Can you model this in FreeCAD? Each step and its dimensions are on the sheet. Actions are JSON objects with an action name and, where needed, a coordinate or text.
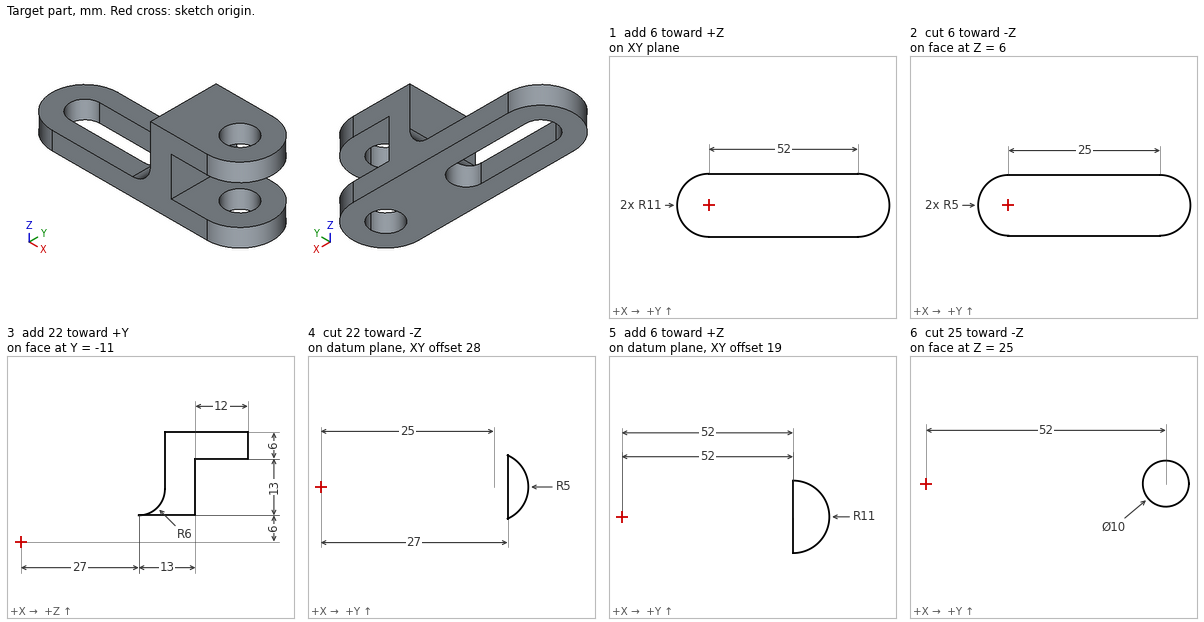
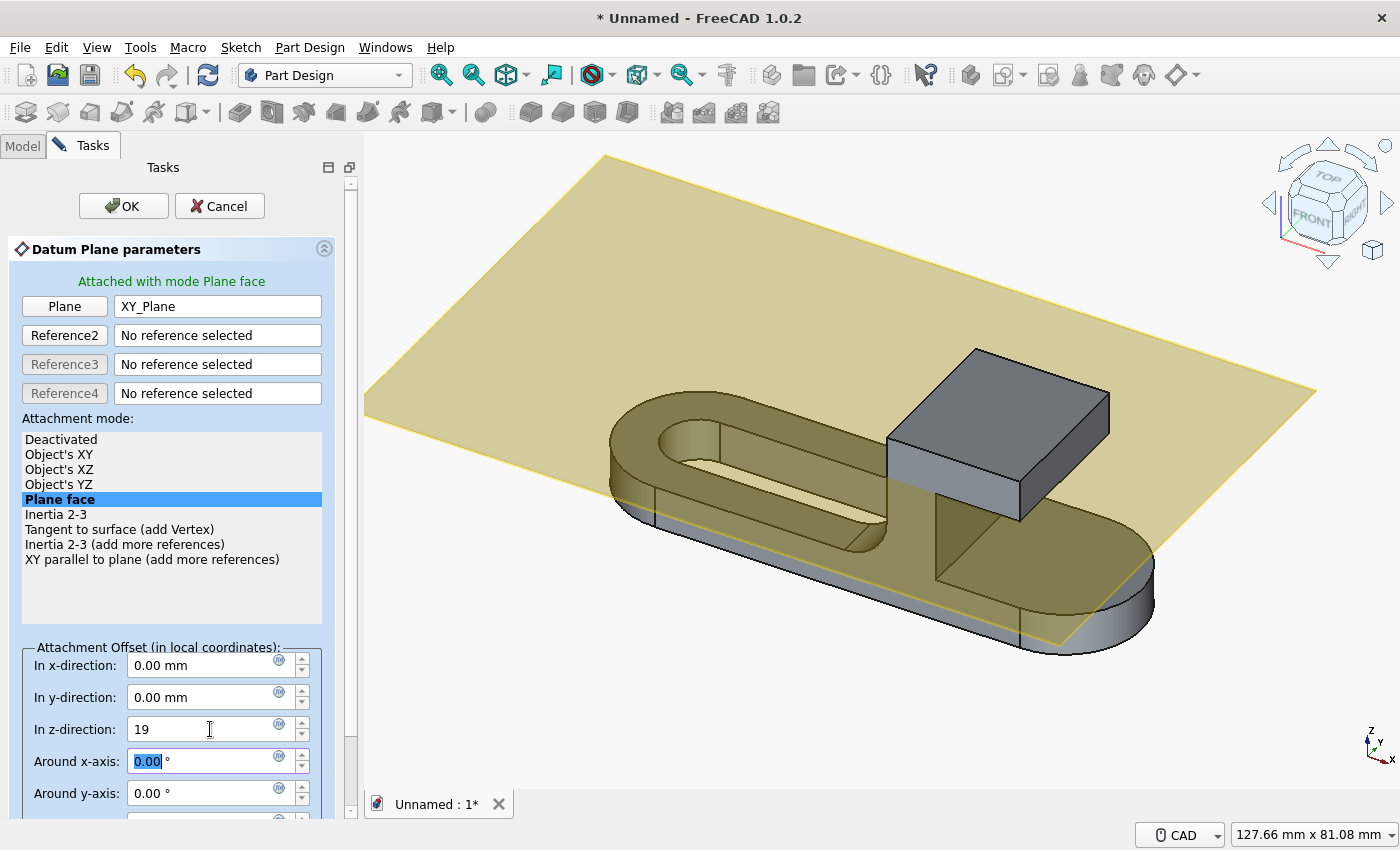
{"action": "left_click", "coordinate": [124, 206]}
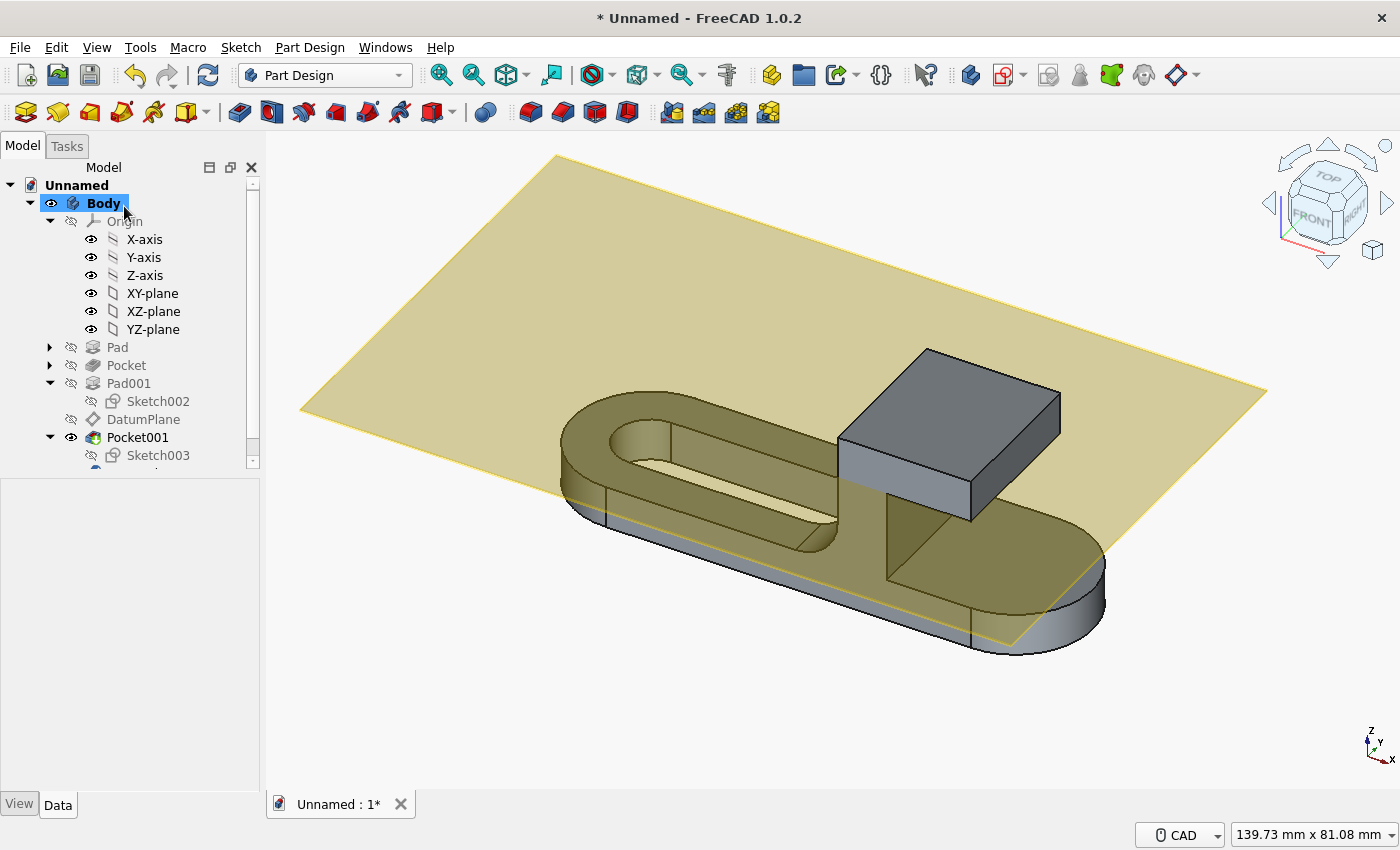
{"action": "scroll", "coordinate": [100, 325], "scroll_direction": "down", "scroll_amount": 3}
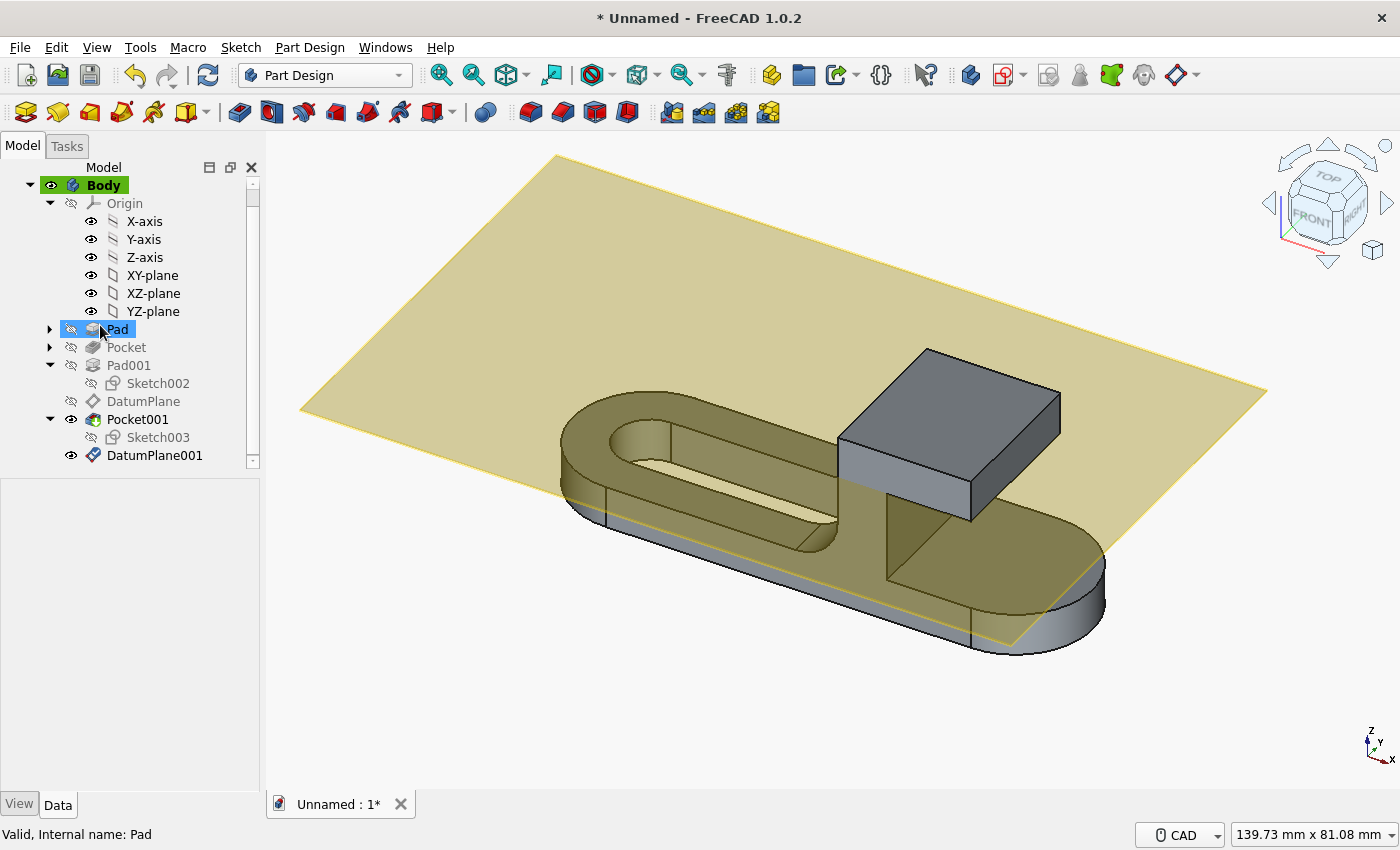
{"action": "left_click", "coordinate": [116, 455]}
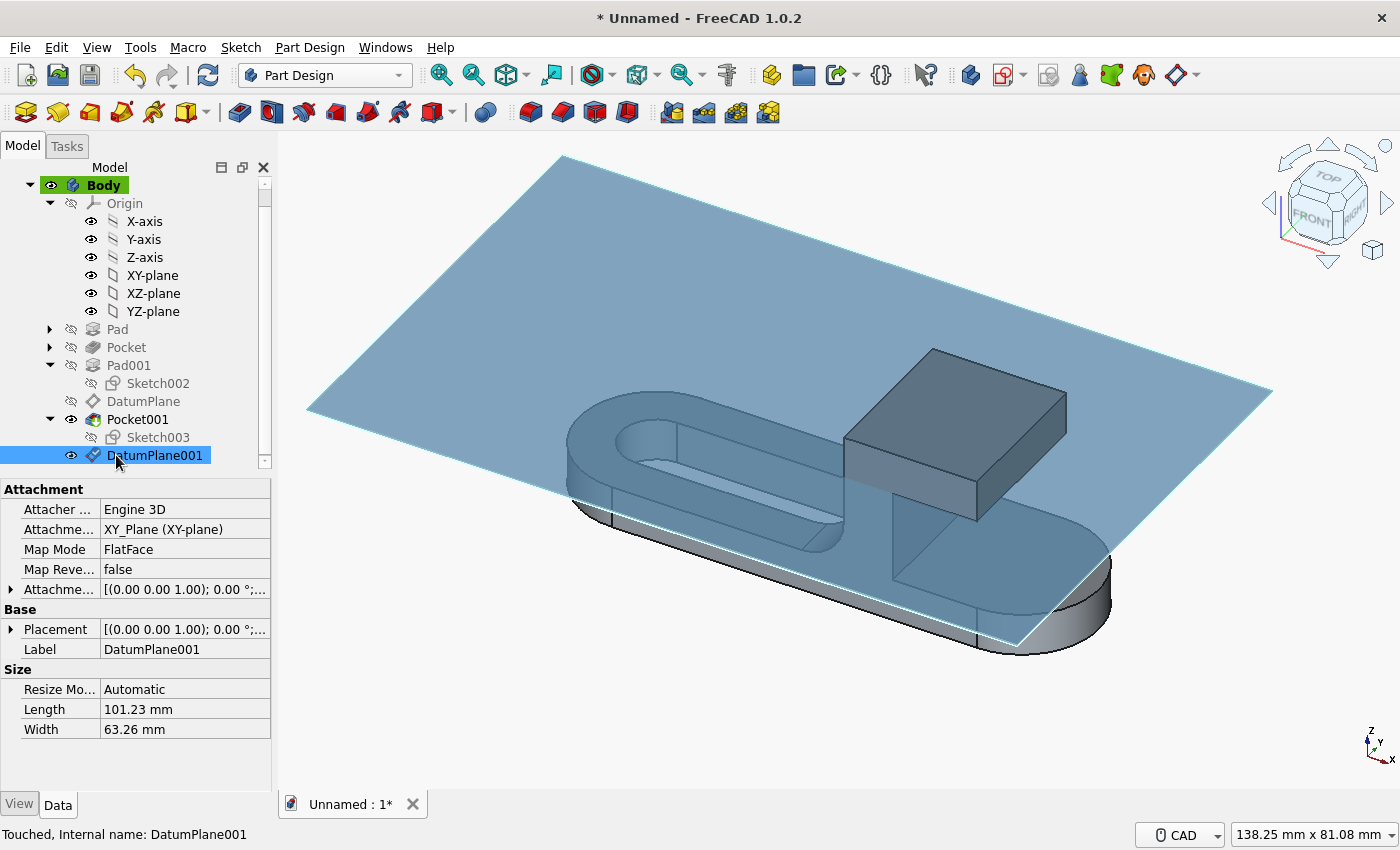
{"action": "left_click", "coordinate": [1004, 76]}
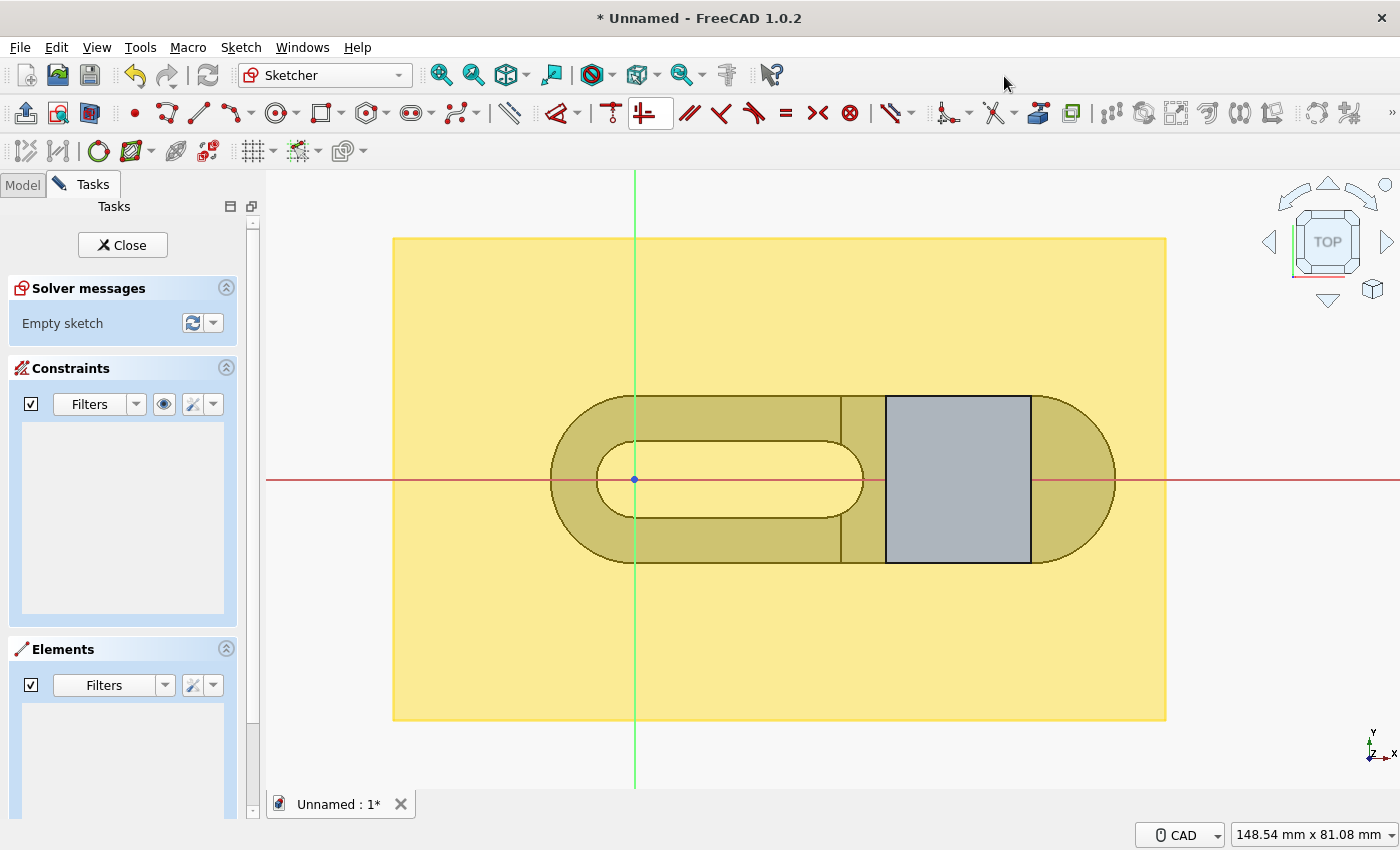
{"action": "left_click", "coordinate": [90, 114]}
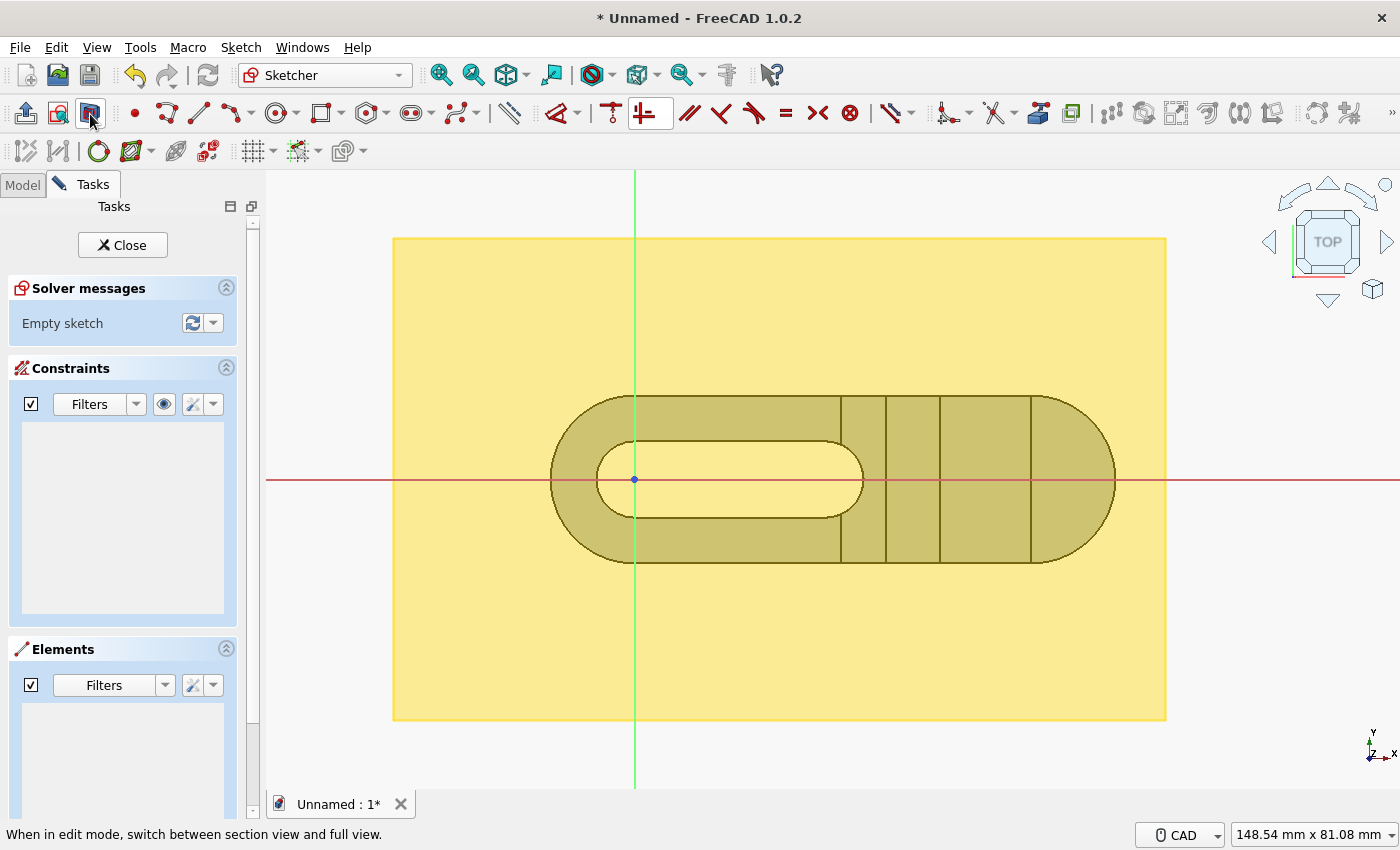
{"action": "scroll", "coordinate": [1235, 480], "scroll_direction": "up", "scroll_amount": 4}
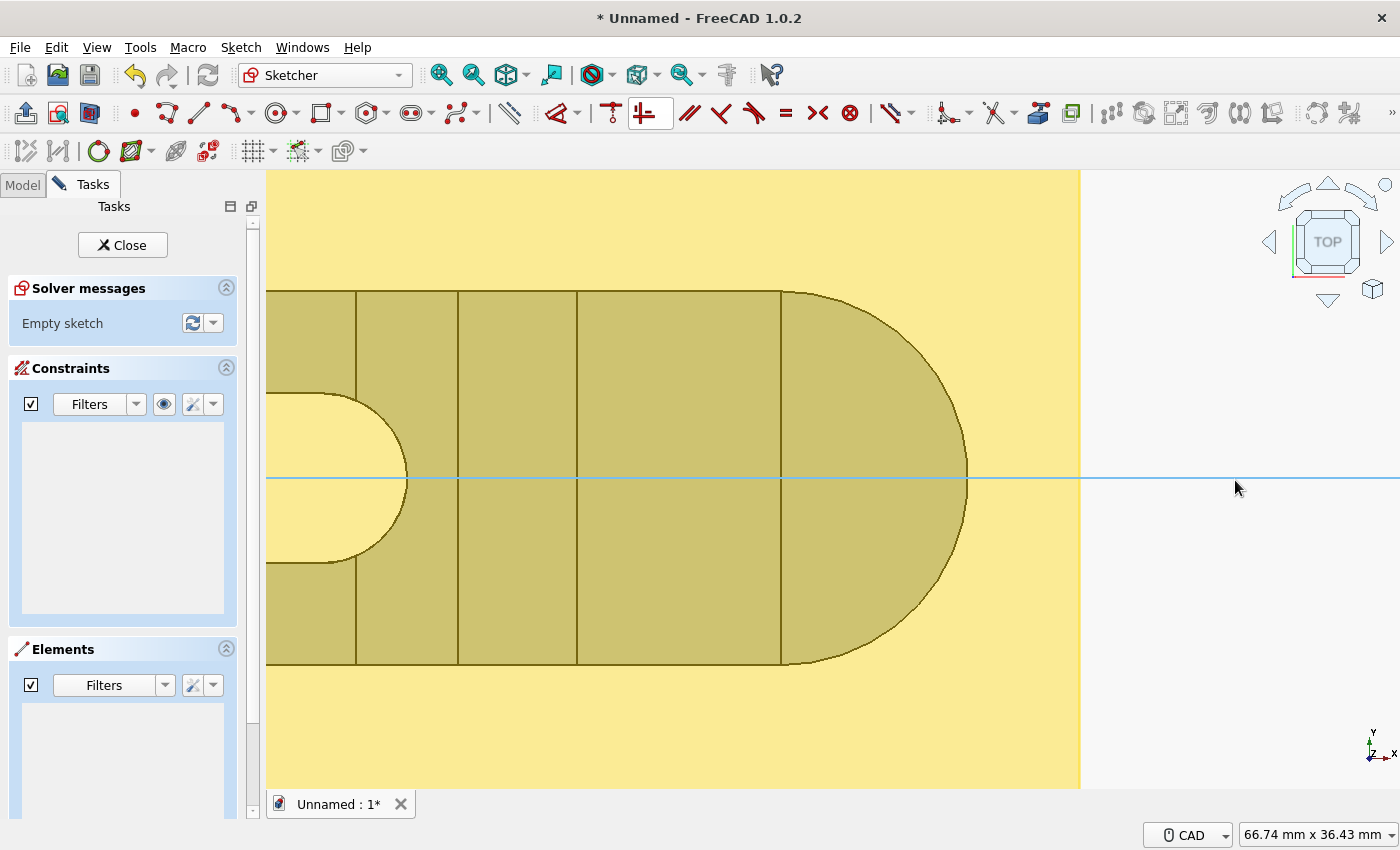
{"action": "key", "text": "g l"}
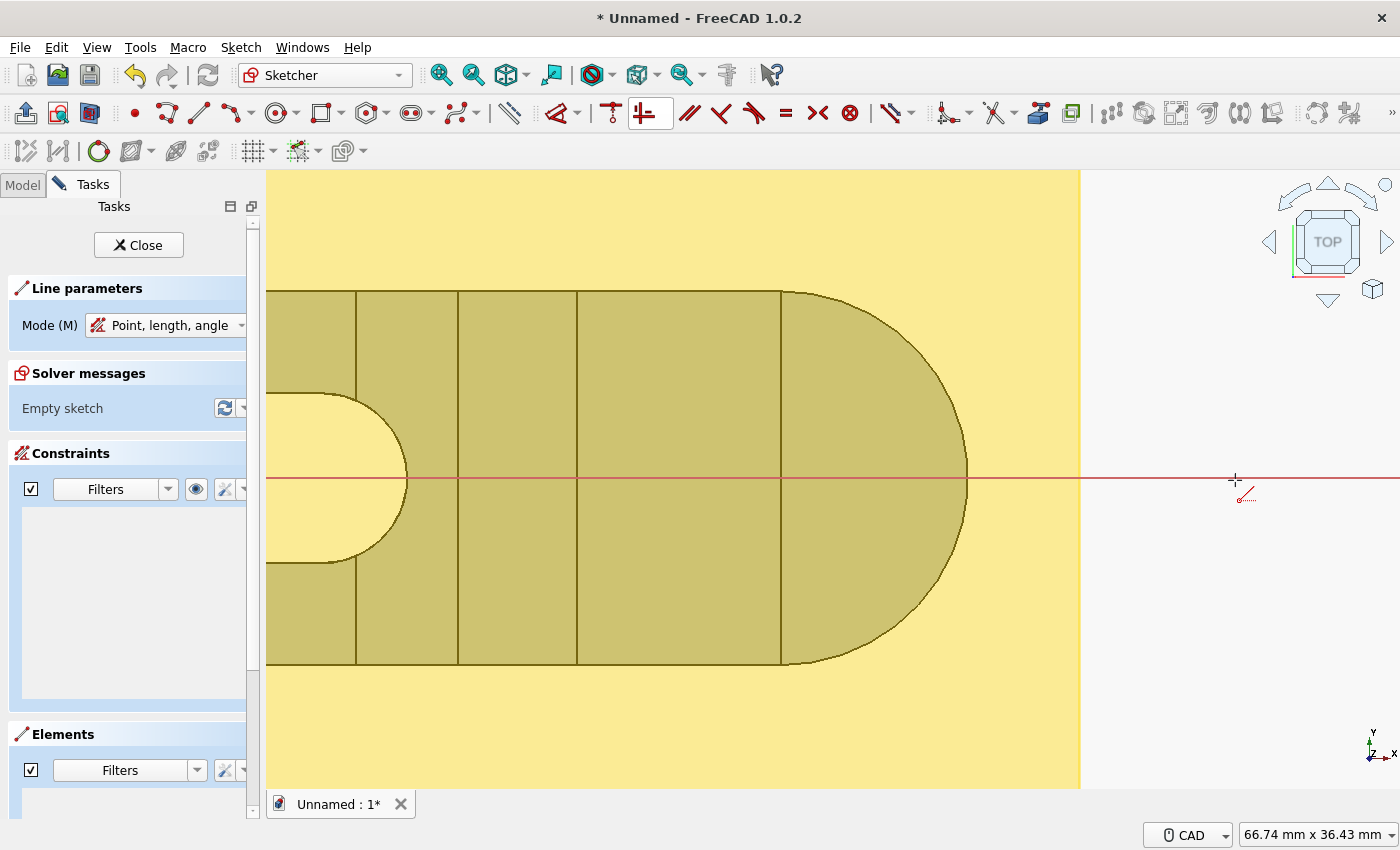
{"action": "left_click", "coordinate": [781, 291]}
{"action": "left_click", "coordinate": [781, 665]}